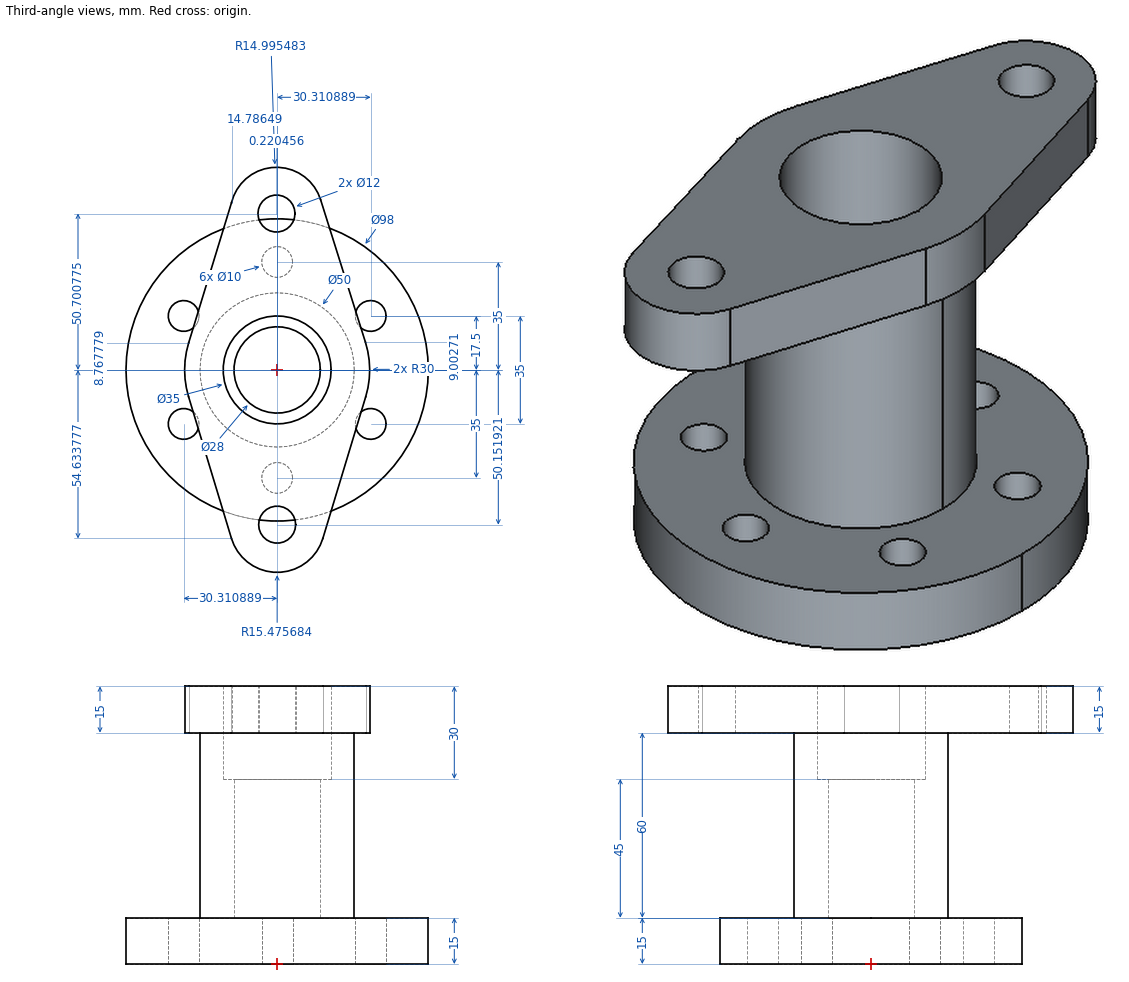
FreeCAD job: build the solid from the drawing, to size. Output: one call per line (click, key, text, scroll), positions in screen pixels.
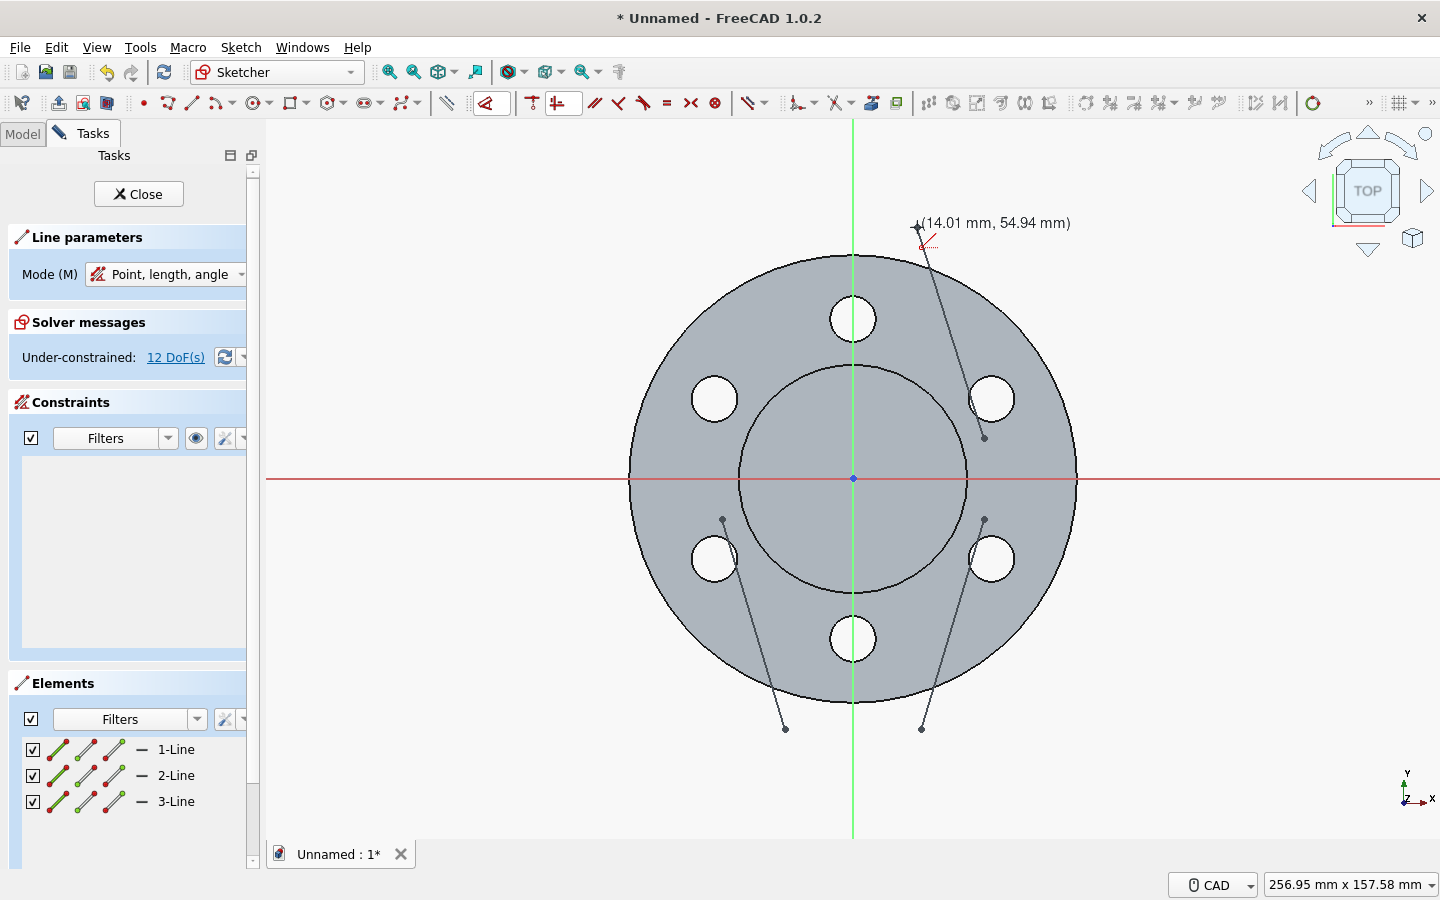
click(785, 231)
click(722, 439)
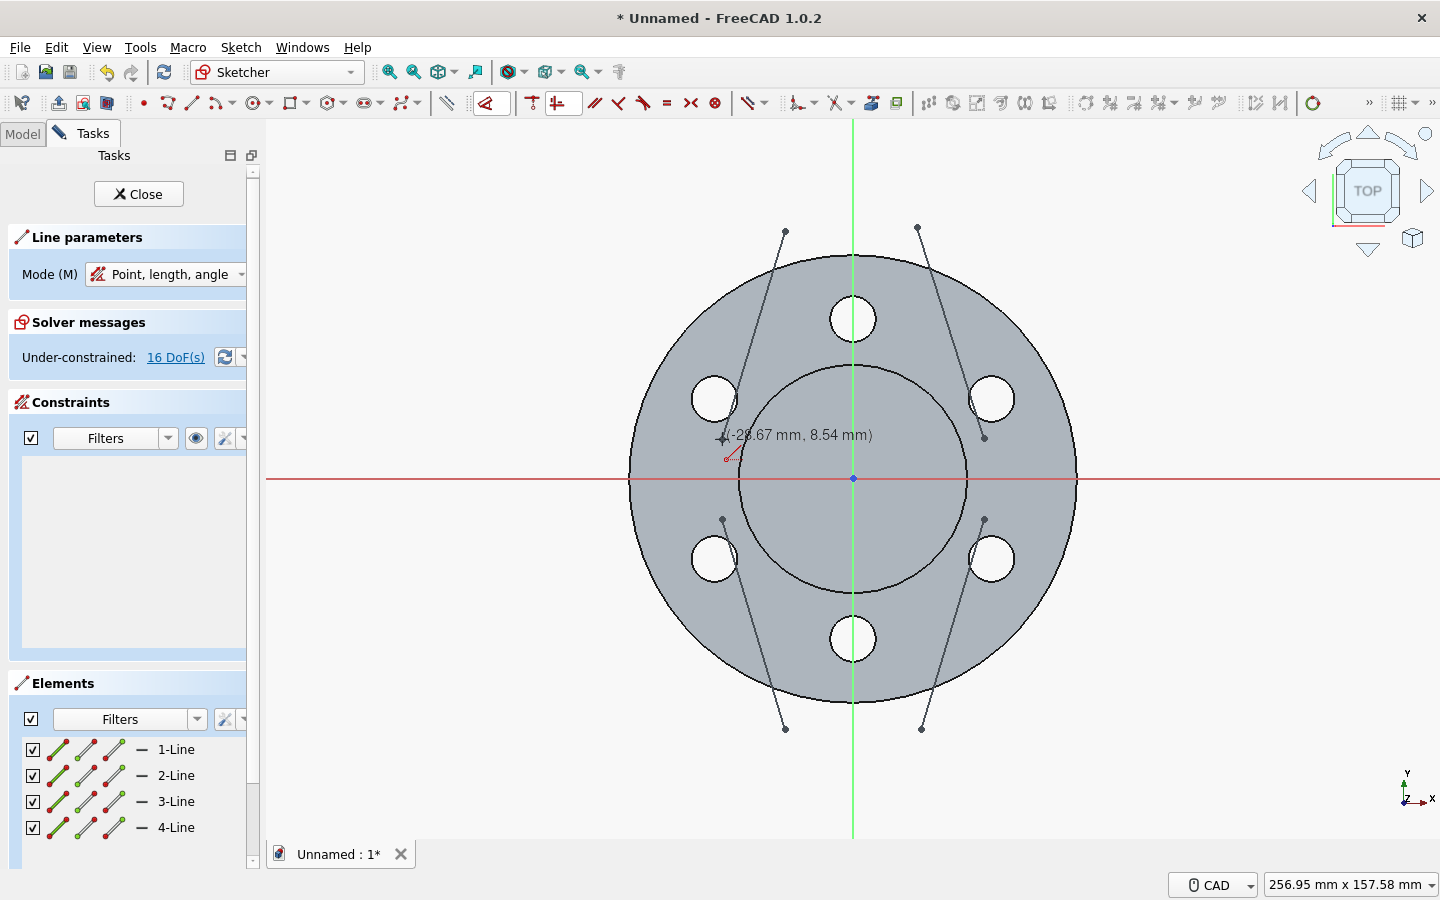
click(234, 104)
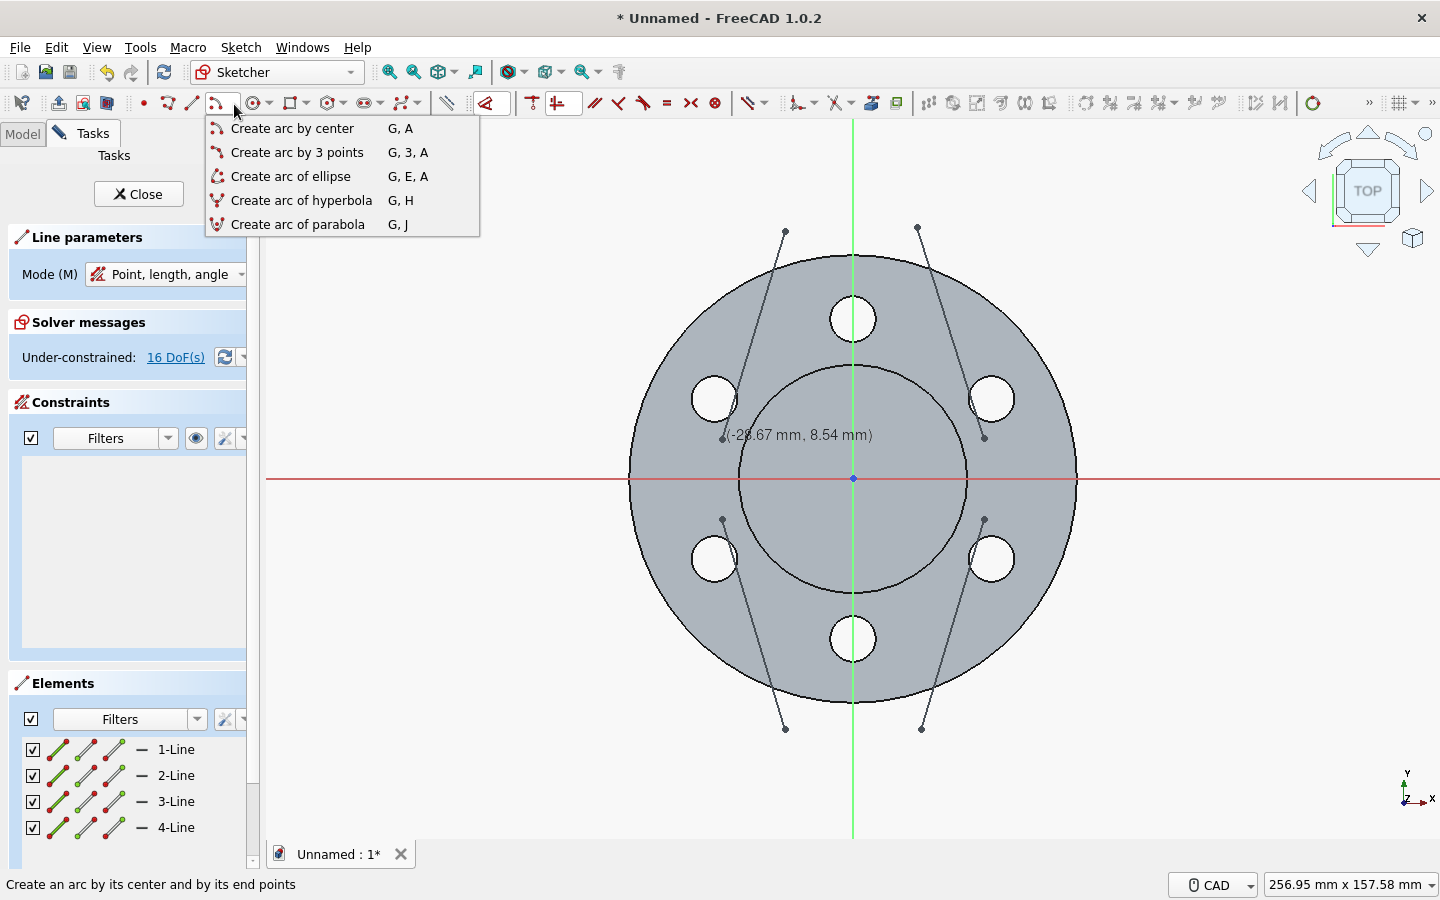
click(342, 152)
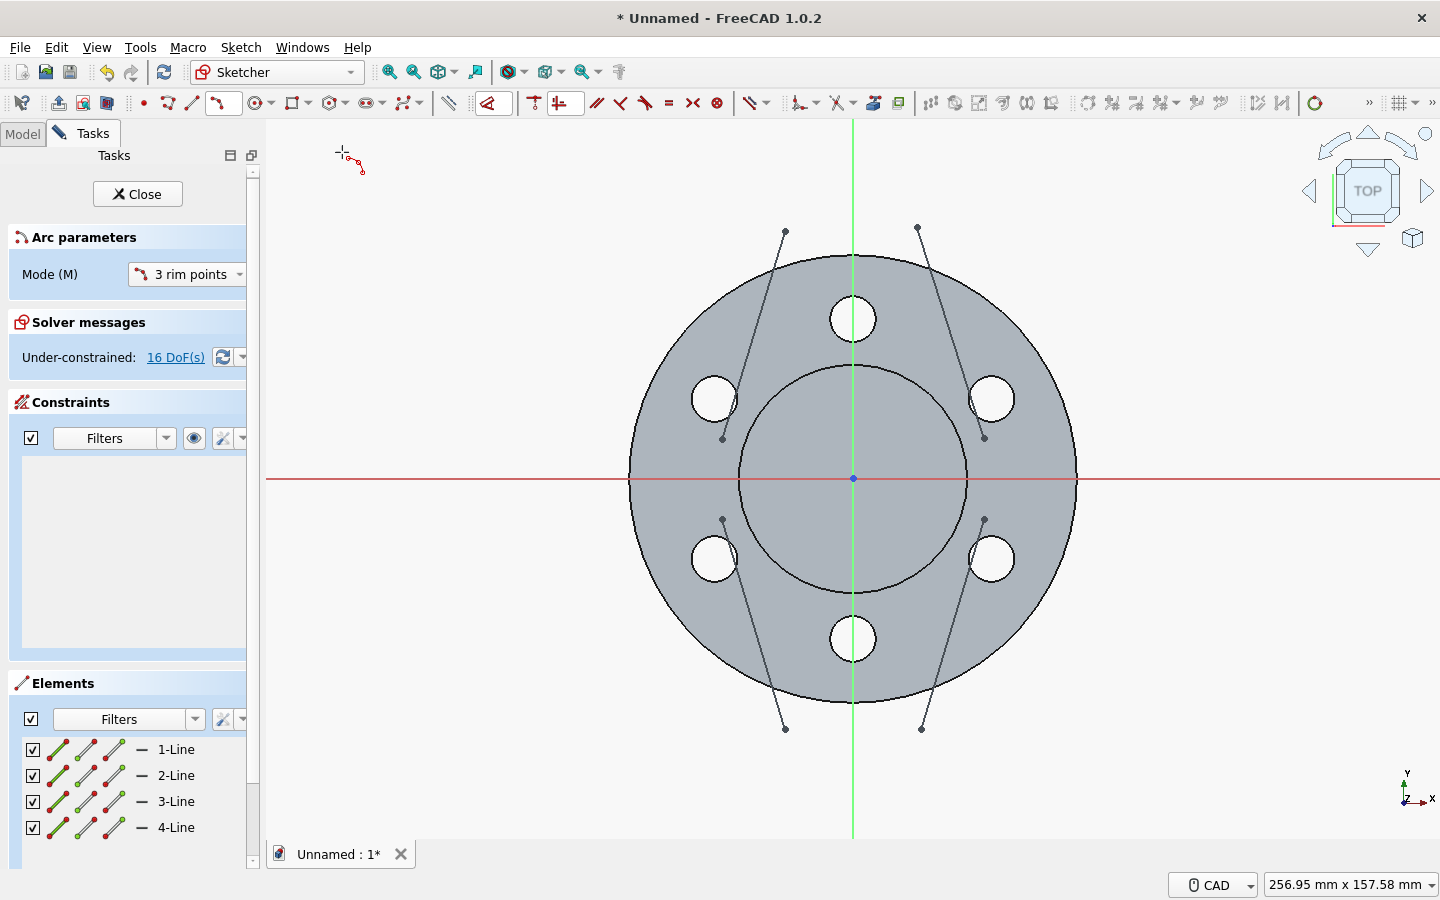
click(785, 730)
click(921, 730)
click(835, 777)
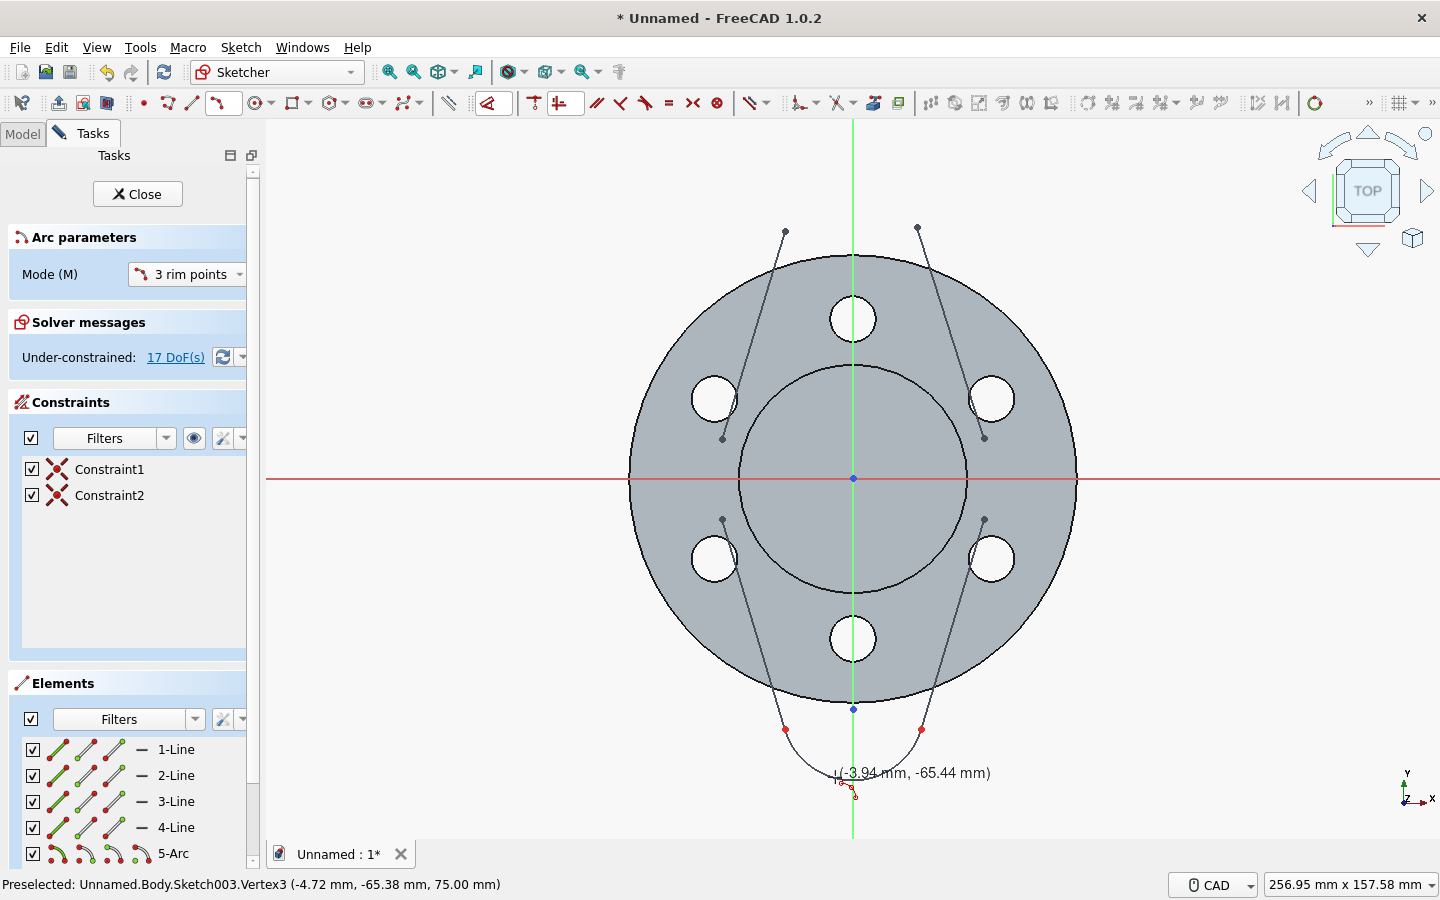
click(984, 520)
click(984, 439)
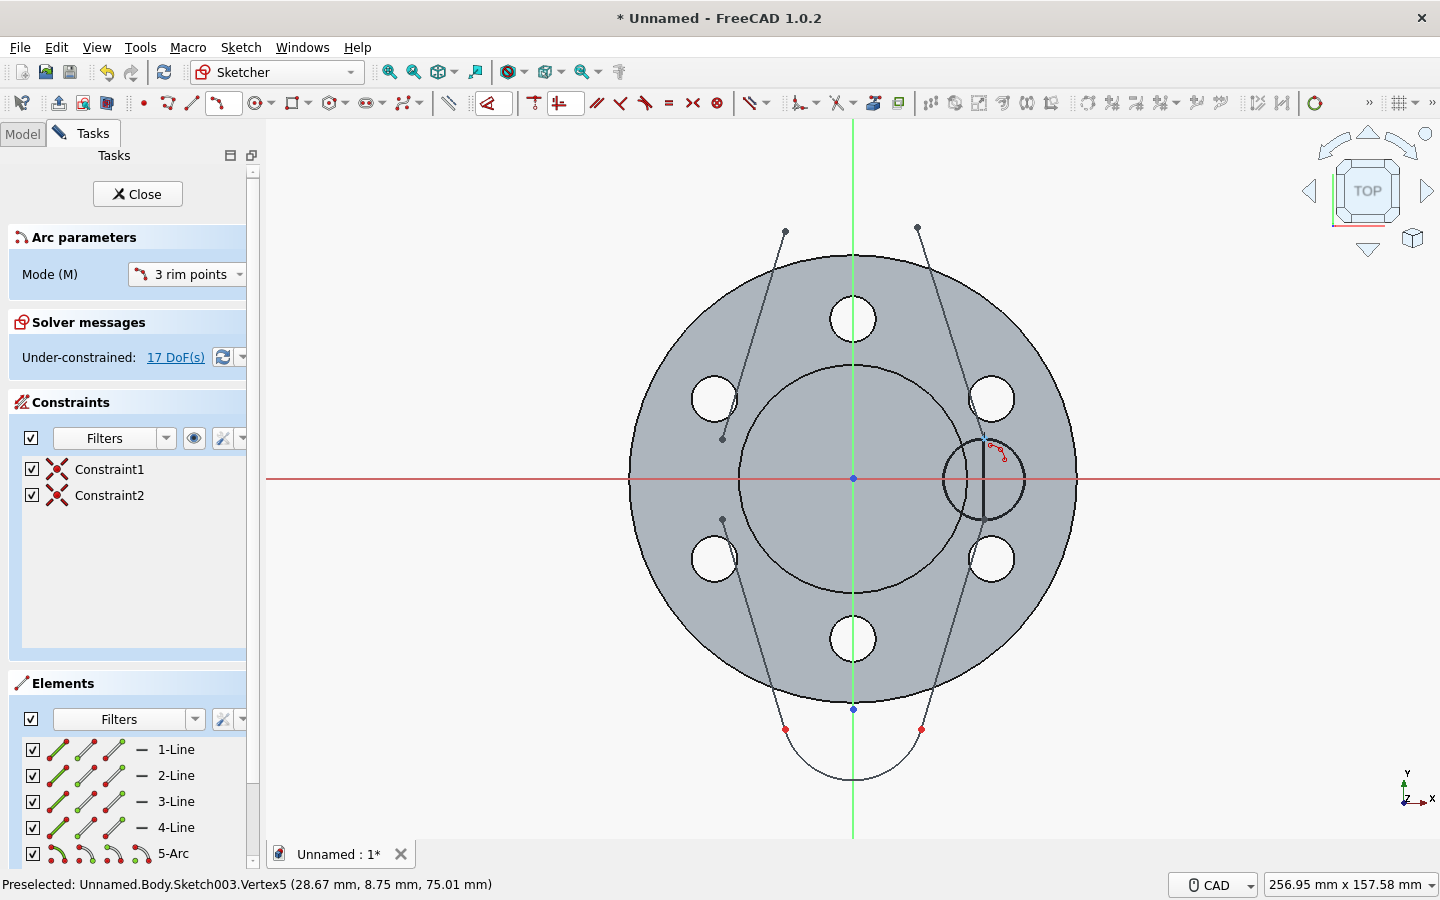
scroll(990, 470, up, 5)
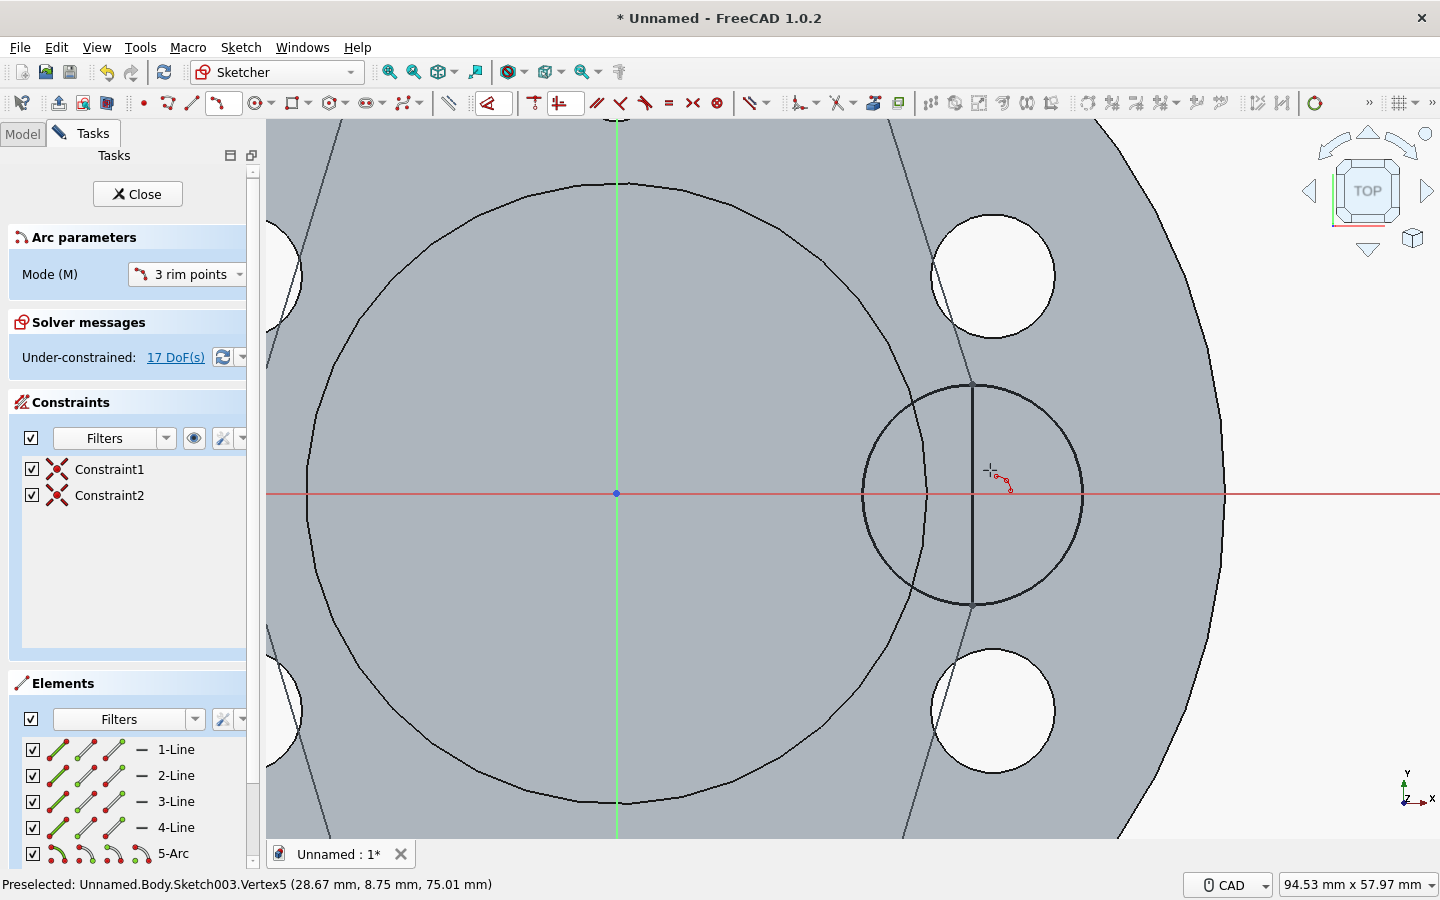
click(988, 469)